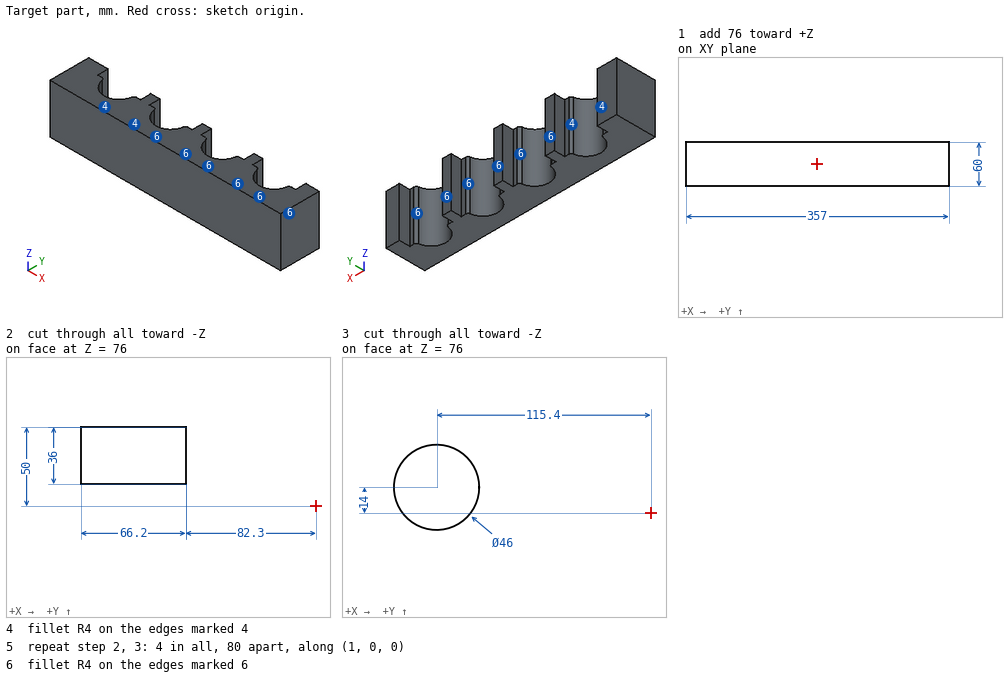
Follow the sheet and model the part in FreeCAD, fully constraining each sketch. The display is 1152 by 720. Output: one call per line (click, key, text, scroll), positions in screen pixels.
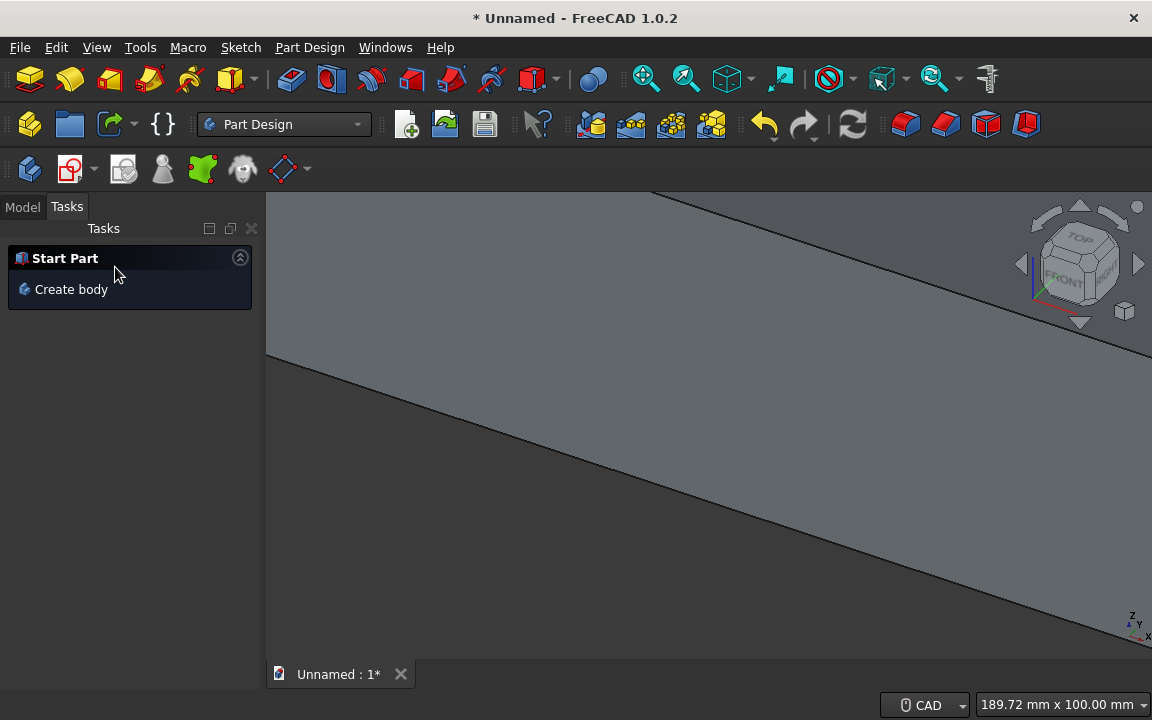
key(v)
key(f)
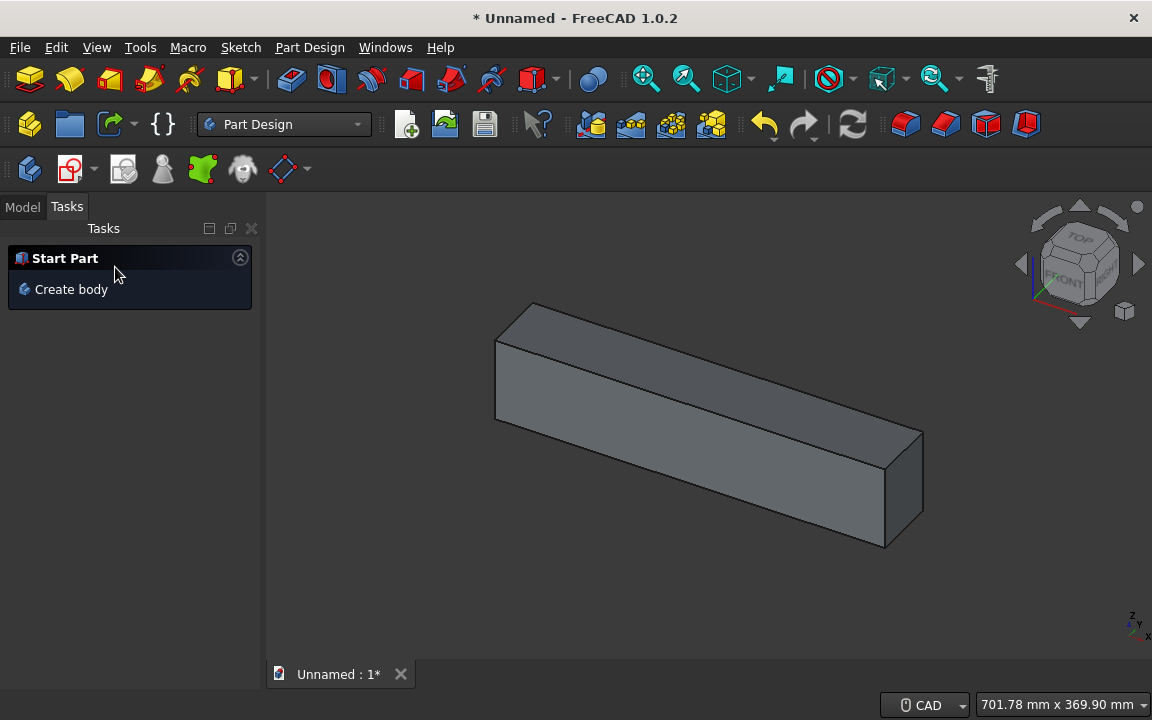
click(821, 422)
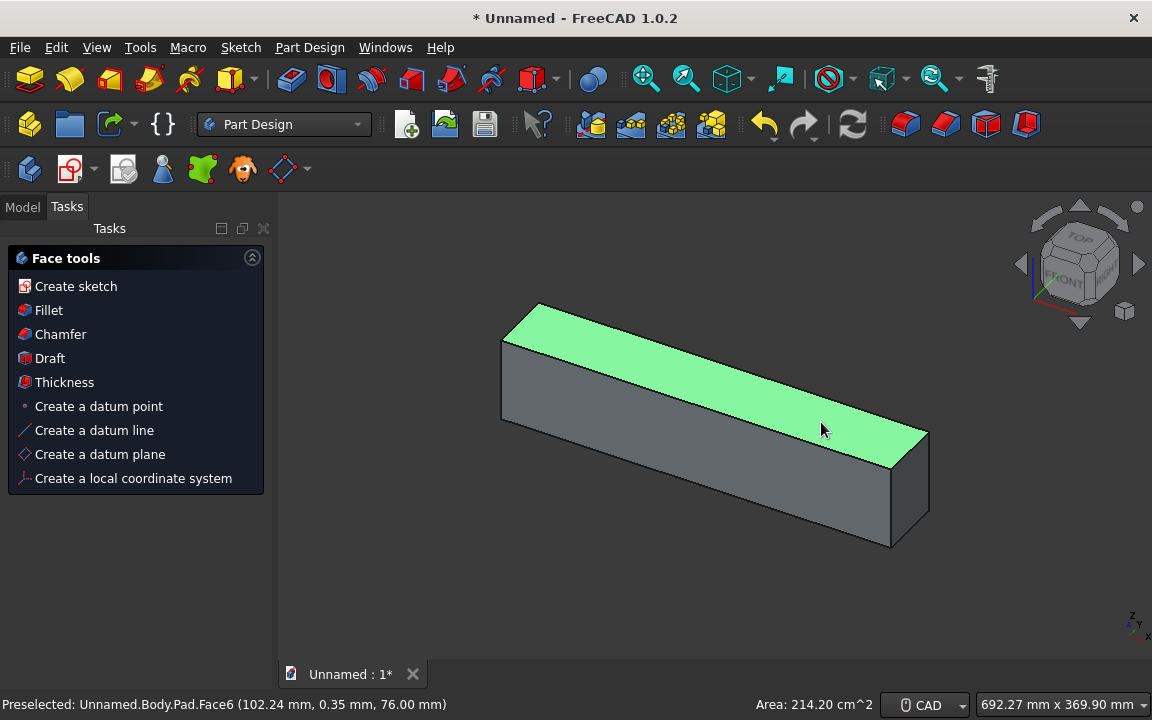
click(70, 170)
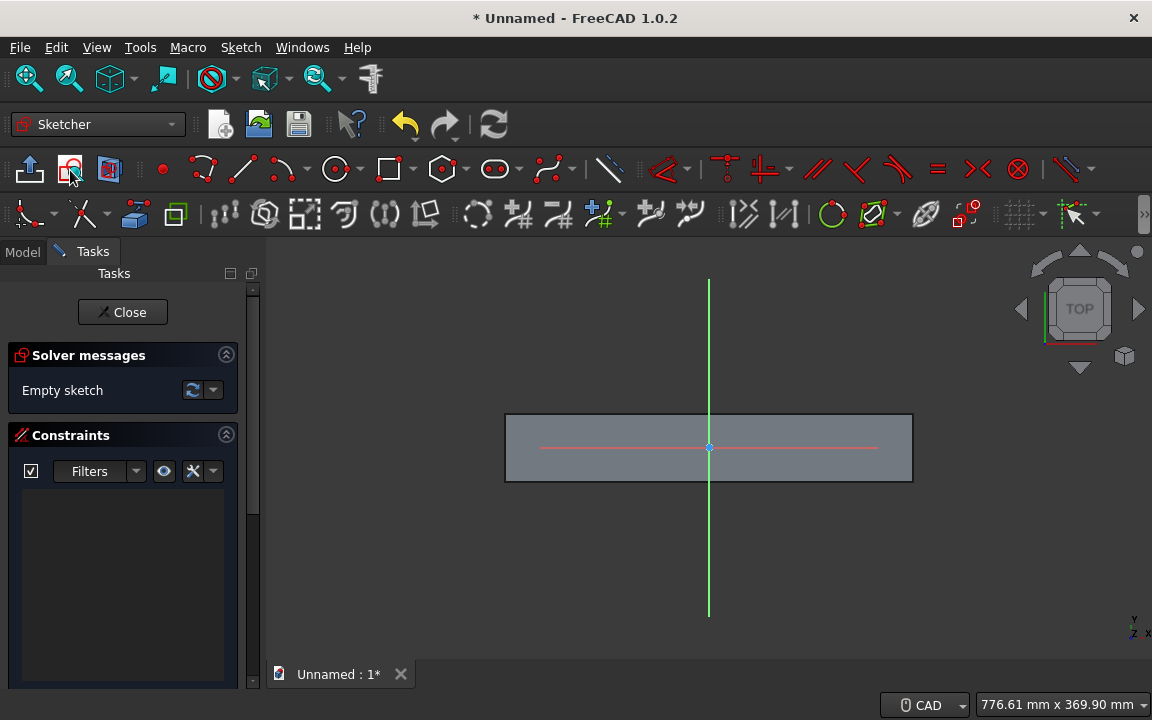
scroll(615, 403, up, 5)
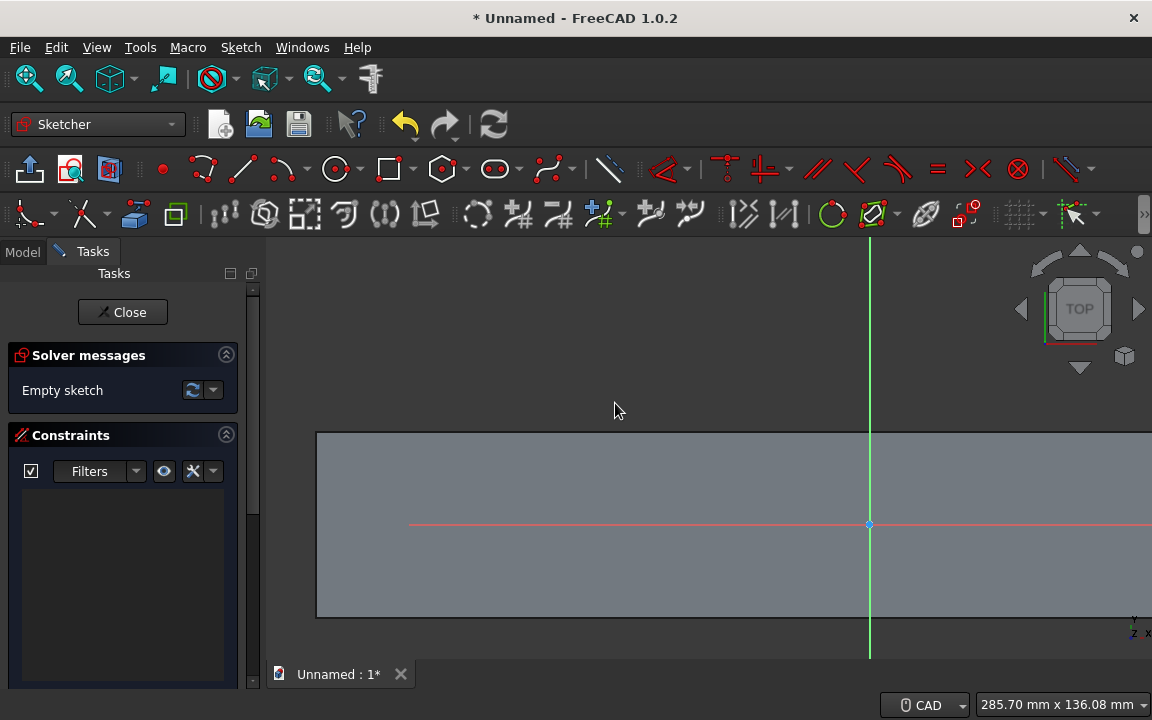
key(g)
key(r)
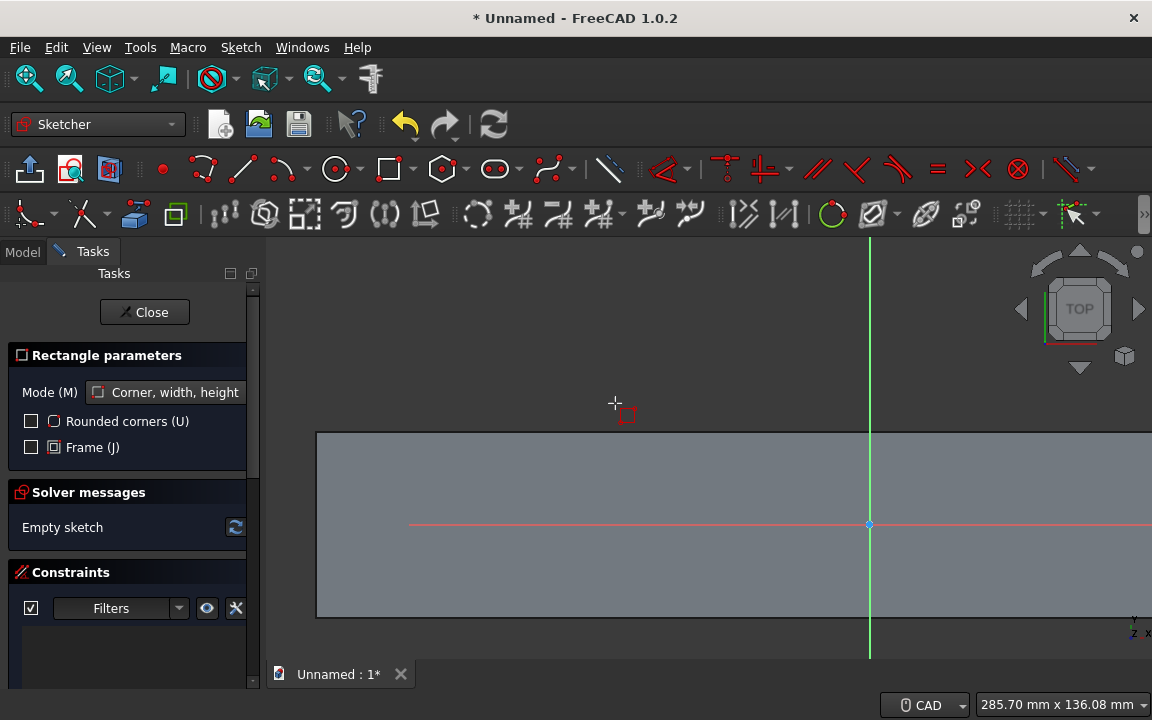
click(409, 370)
move(615, 481)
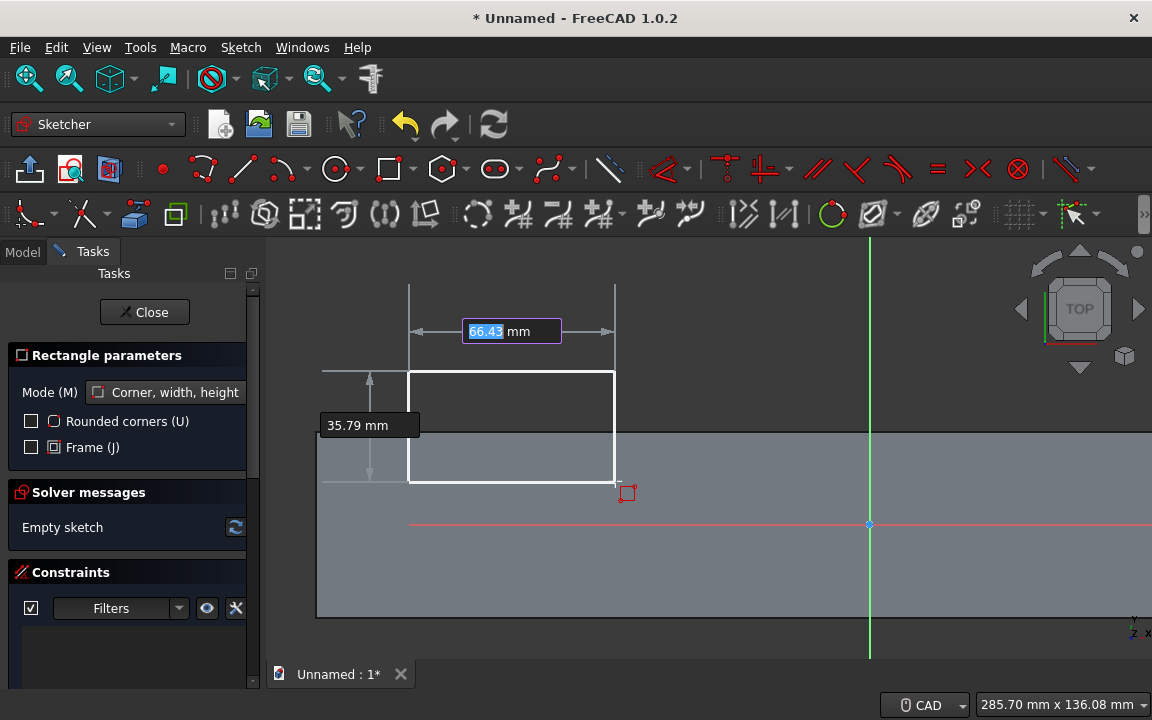
text(66.2)
key(Tab)
text(36)
key(Return)
key(Escape)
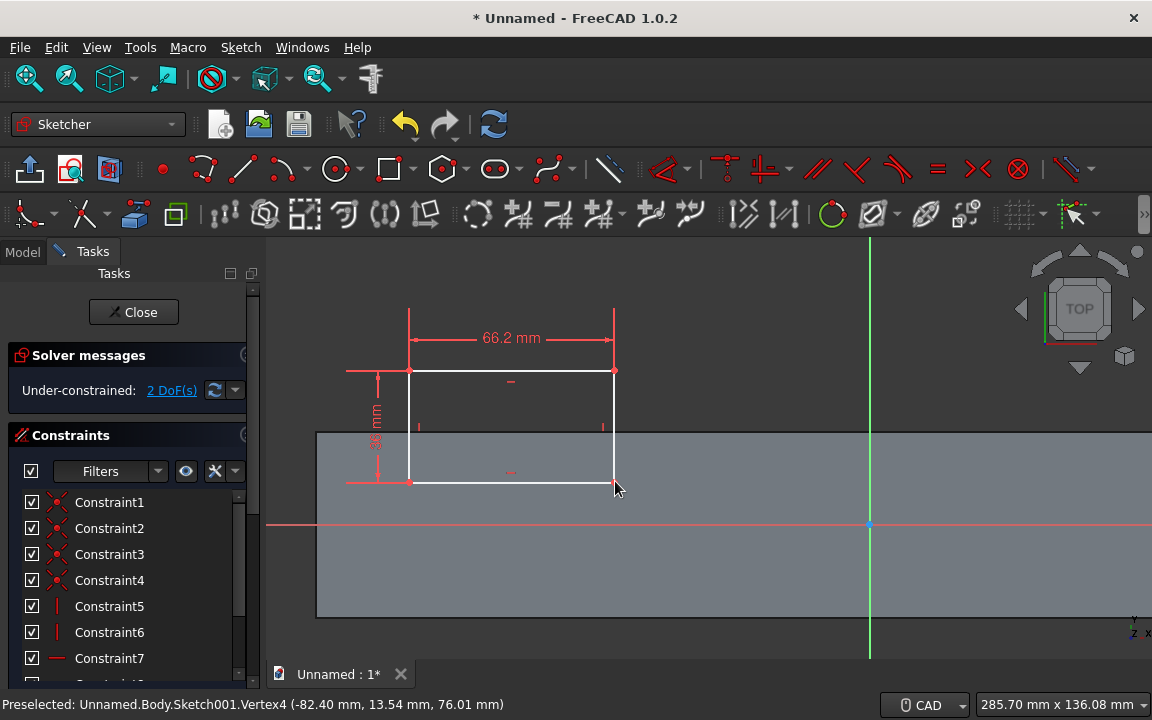
key(d)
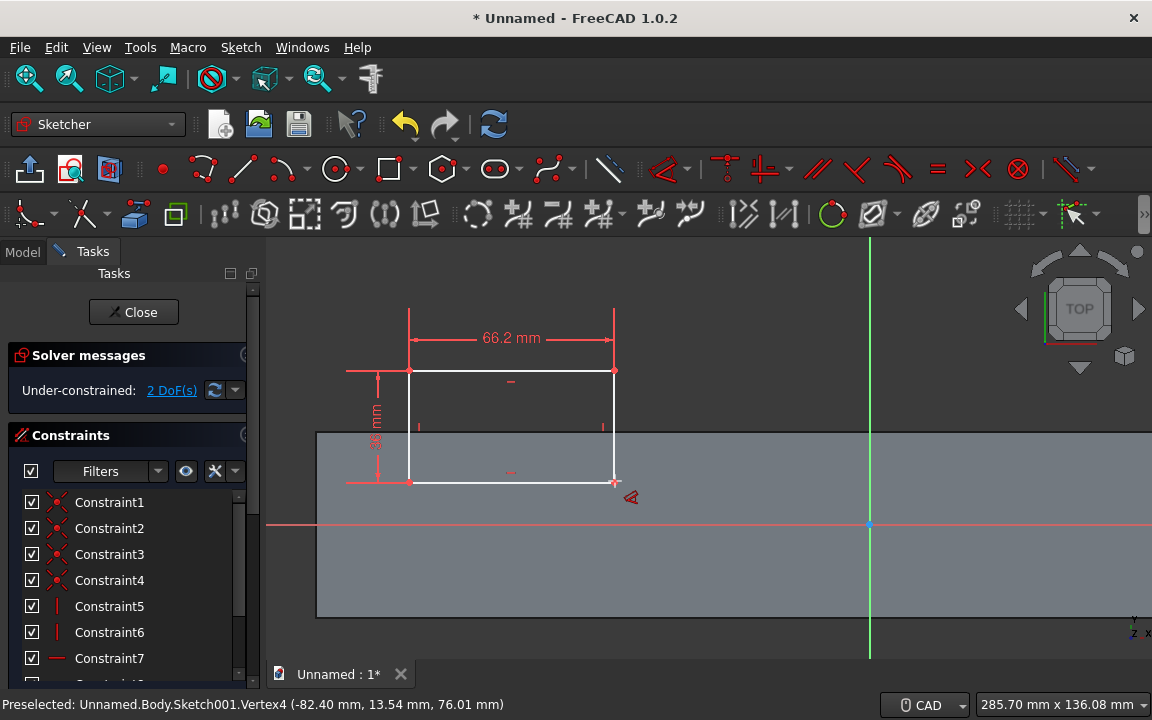
click(409, 371)
click(375, 448)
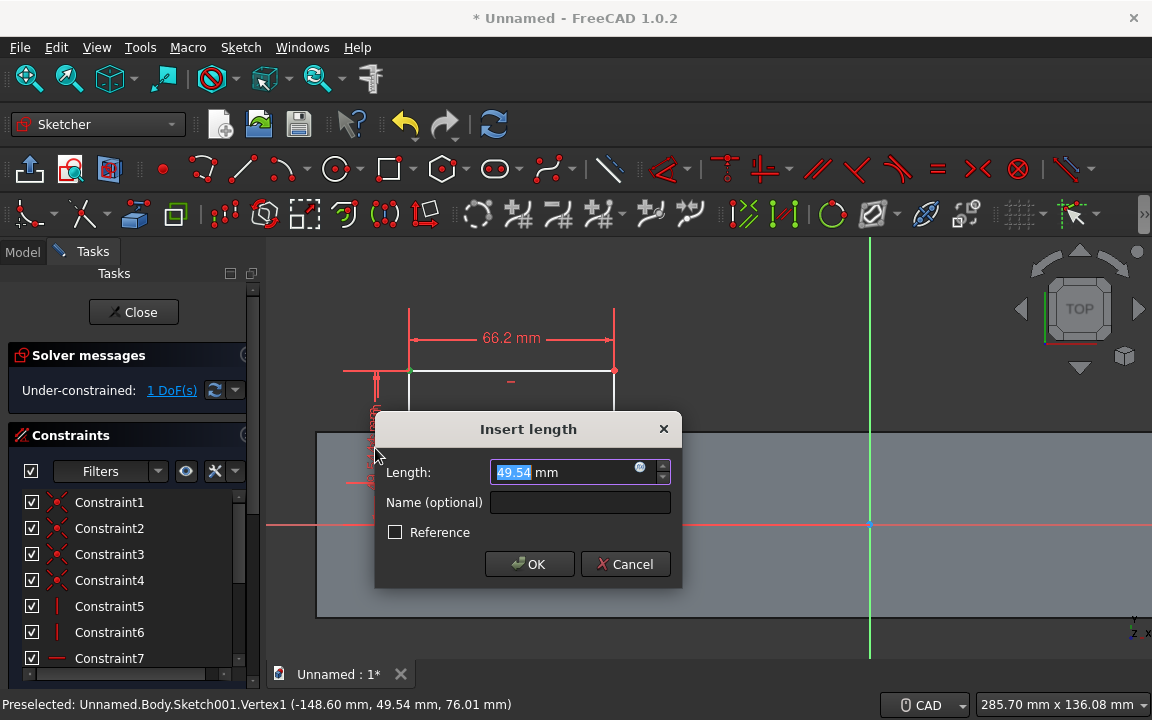
text(50)
key(Return)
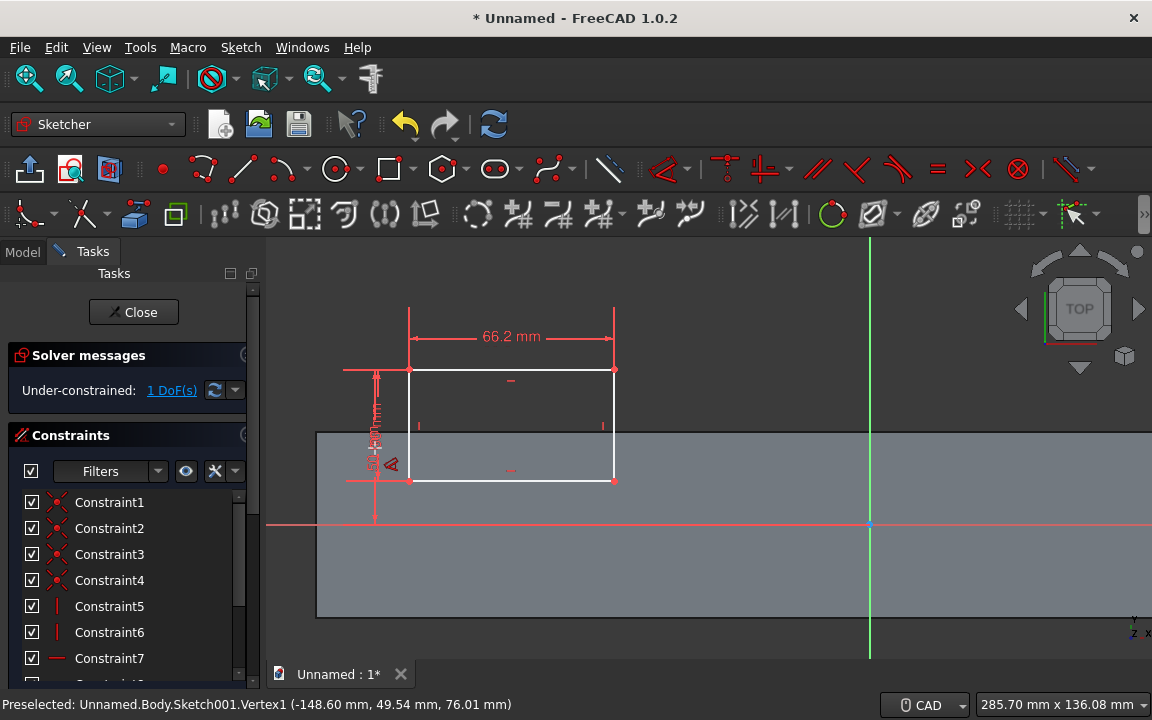
click(614, 481)
click(742, 559)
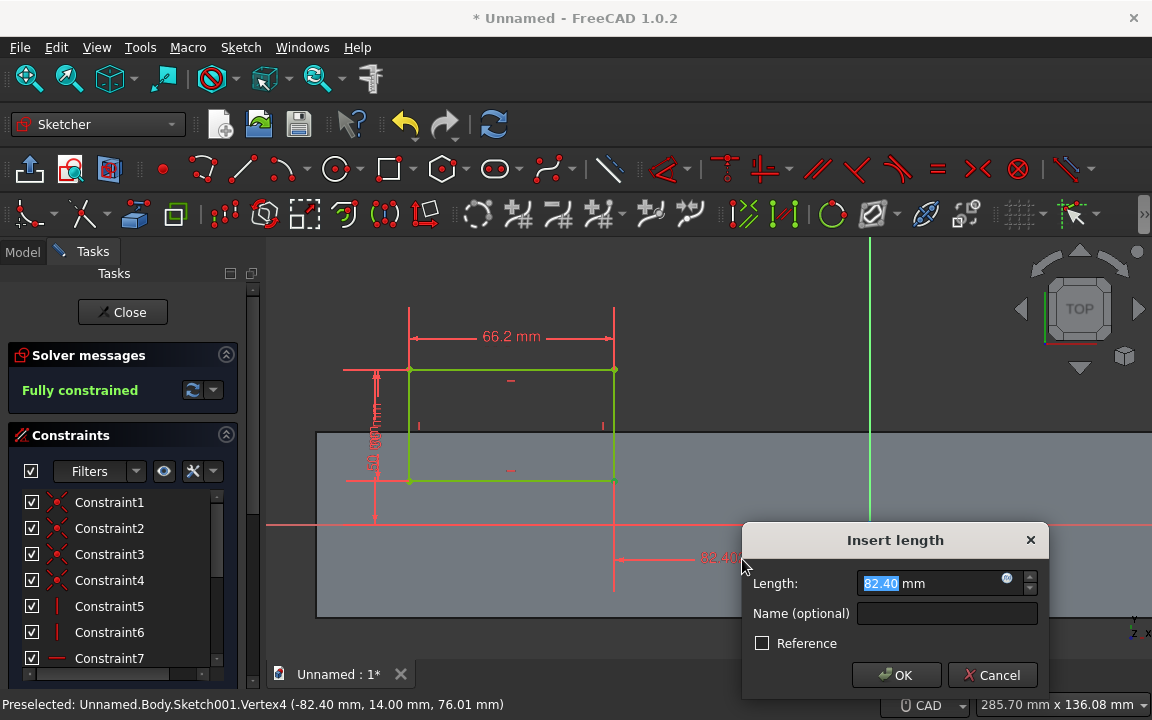
text(82.3)
key(Return)
key(Escape)